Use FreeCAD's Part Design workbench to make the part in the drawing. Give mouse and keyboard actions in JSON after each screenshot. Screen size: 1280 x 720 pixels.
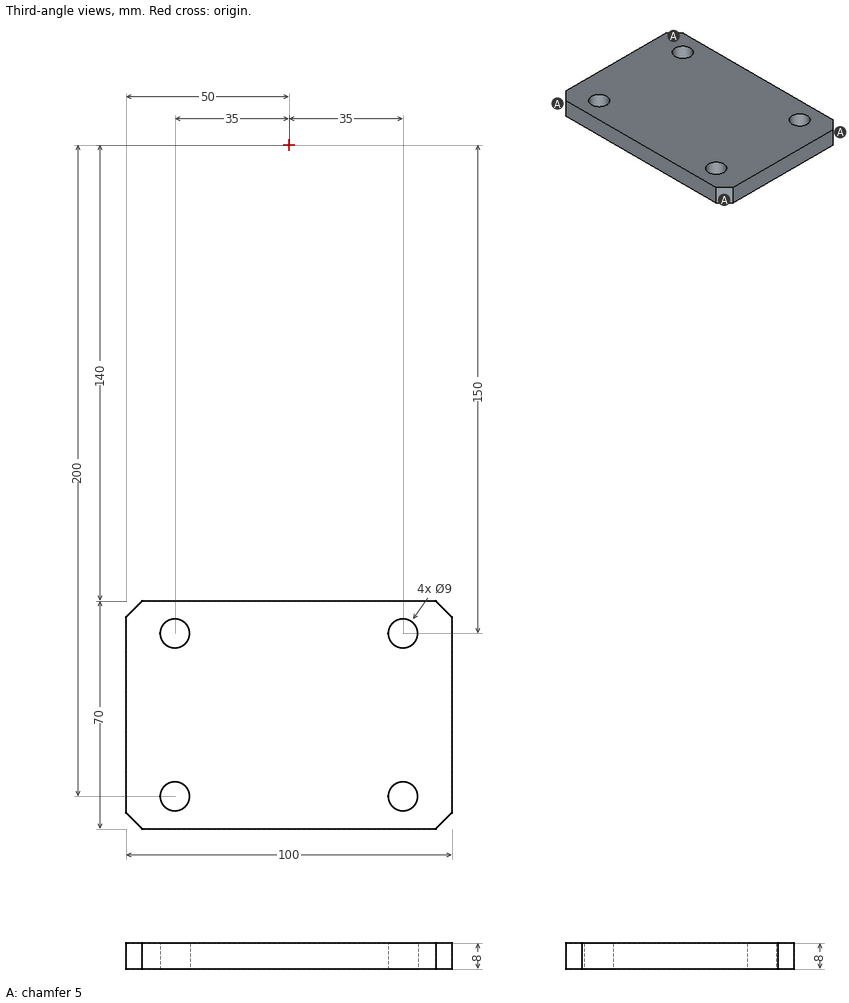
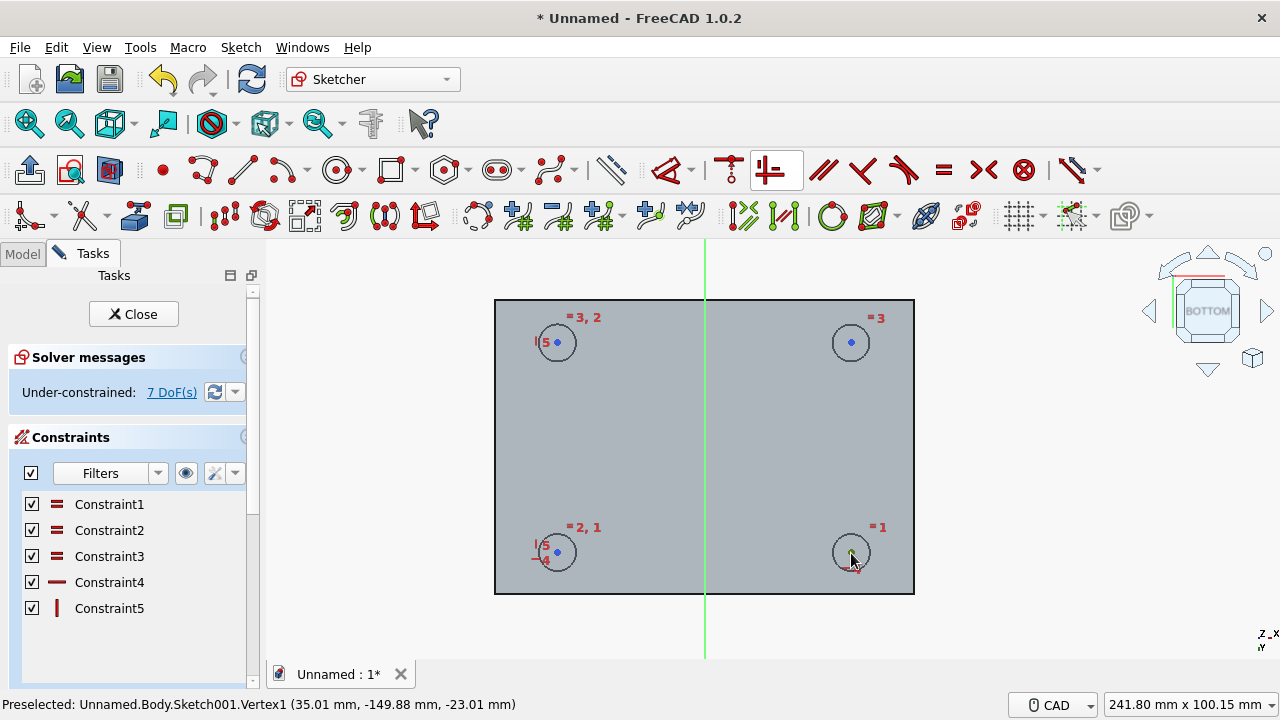
{"action": "left_click", "coordinate": [851, 343]}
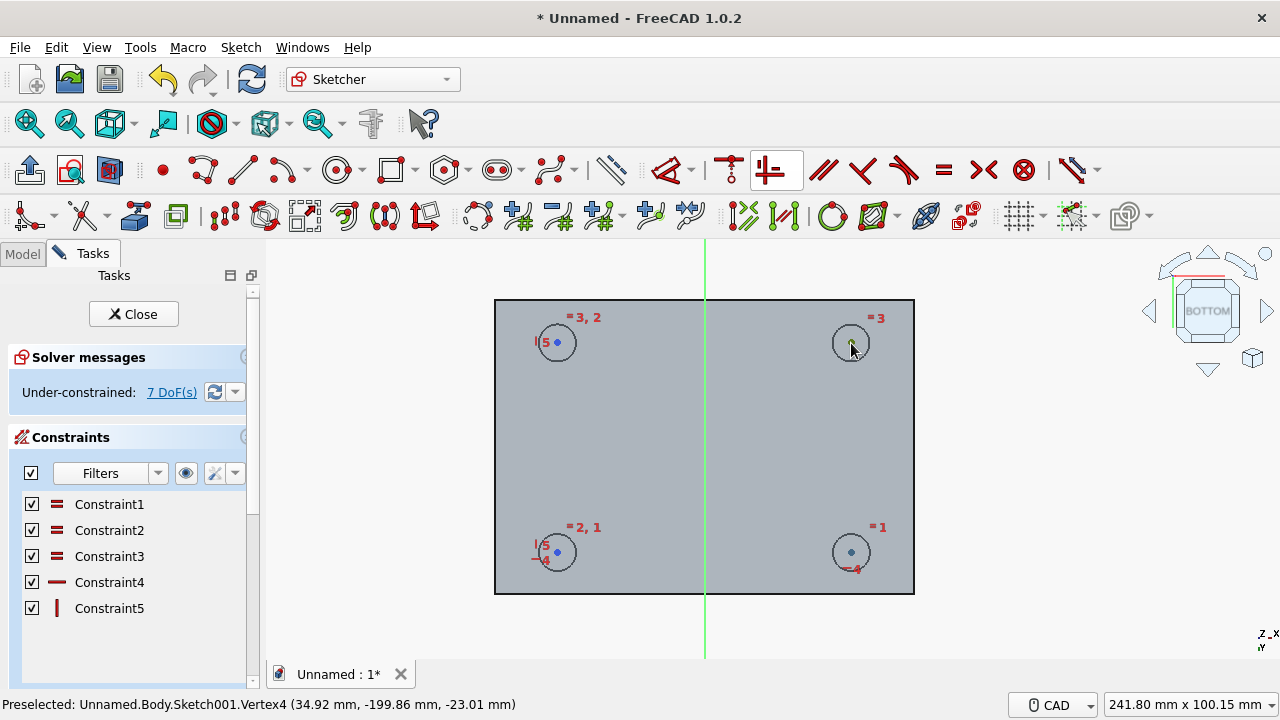
{"action": "left_click", "coordinate": [798, 170]}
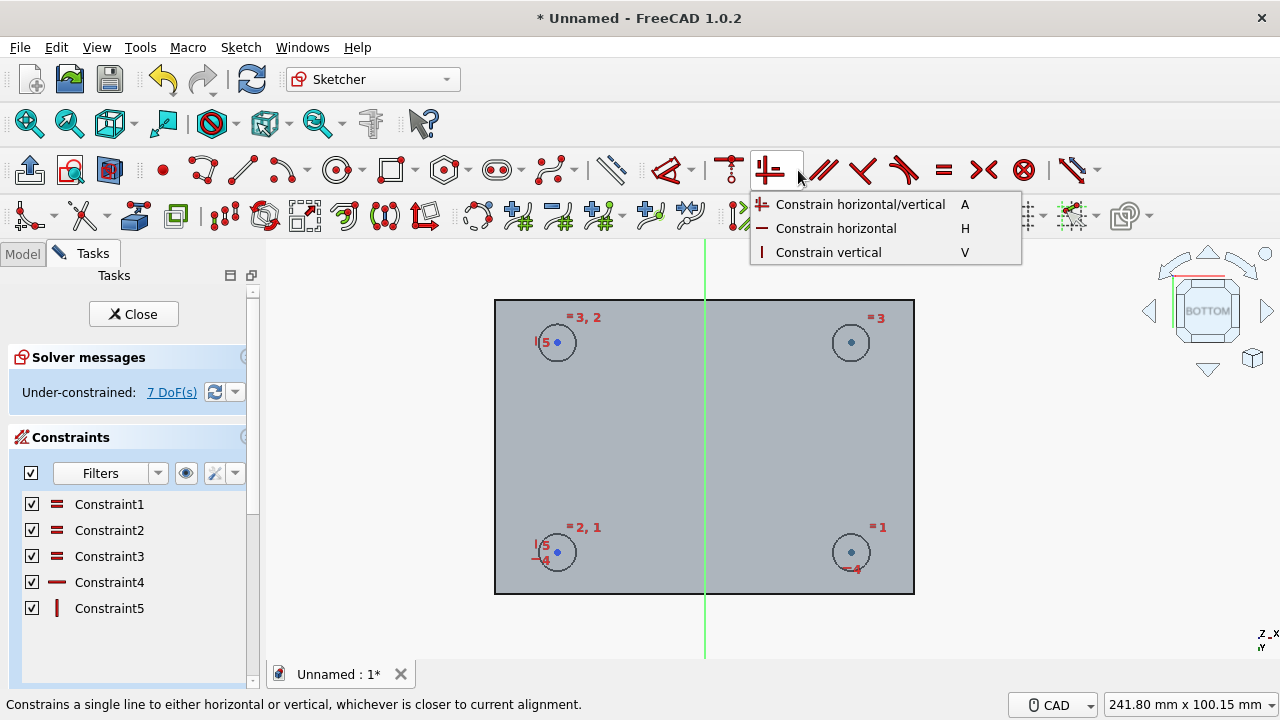
{"action": "left_click", "coordinate": [886, 252]}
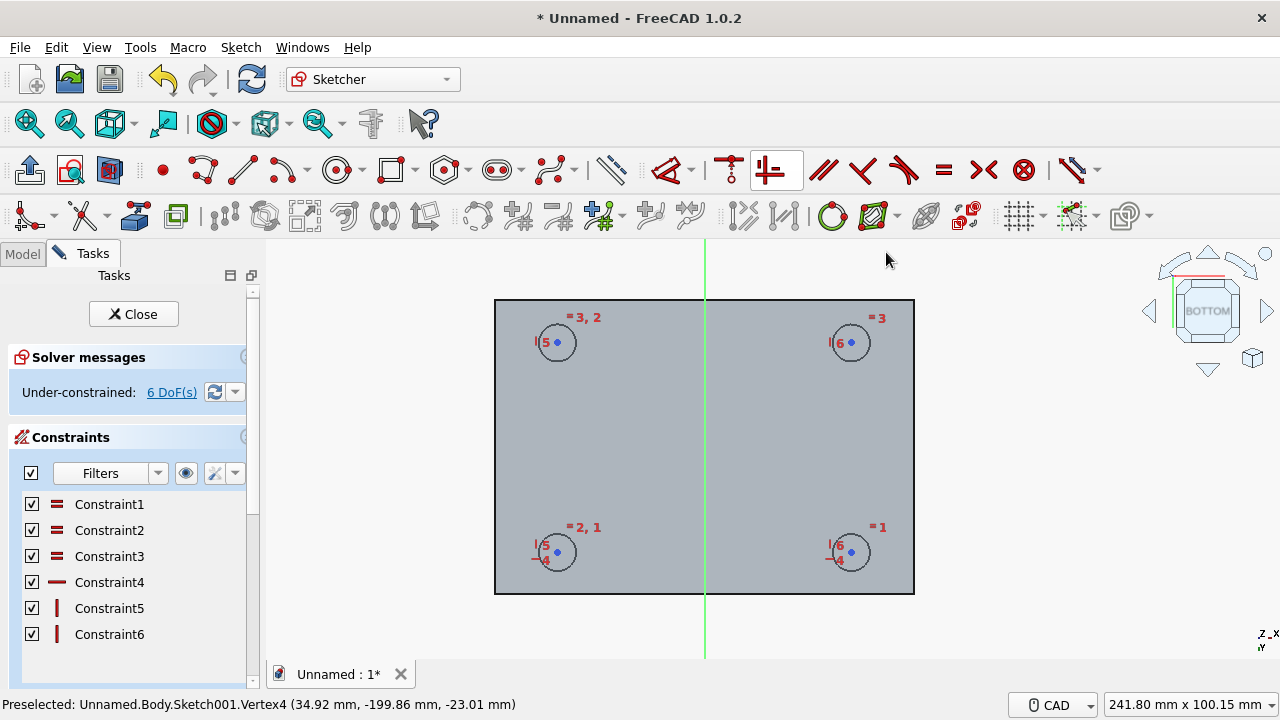
{"action": "left_click", "coordinate": [557, 343]}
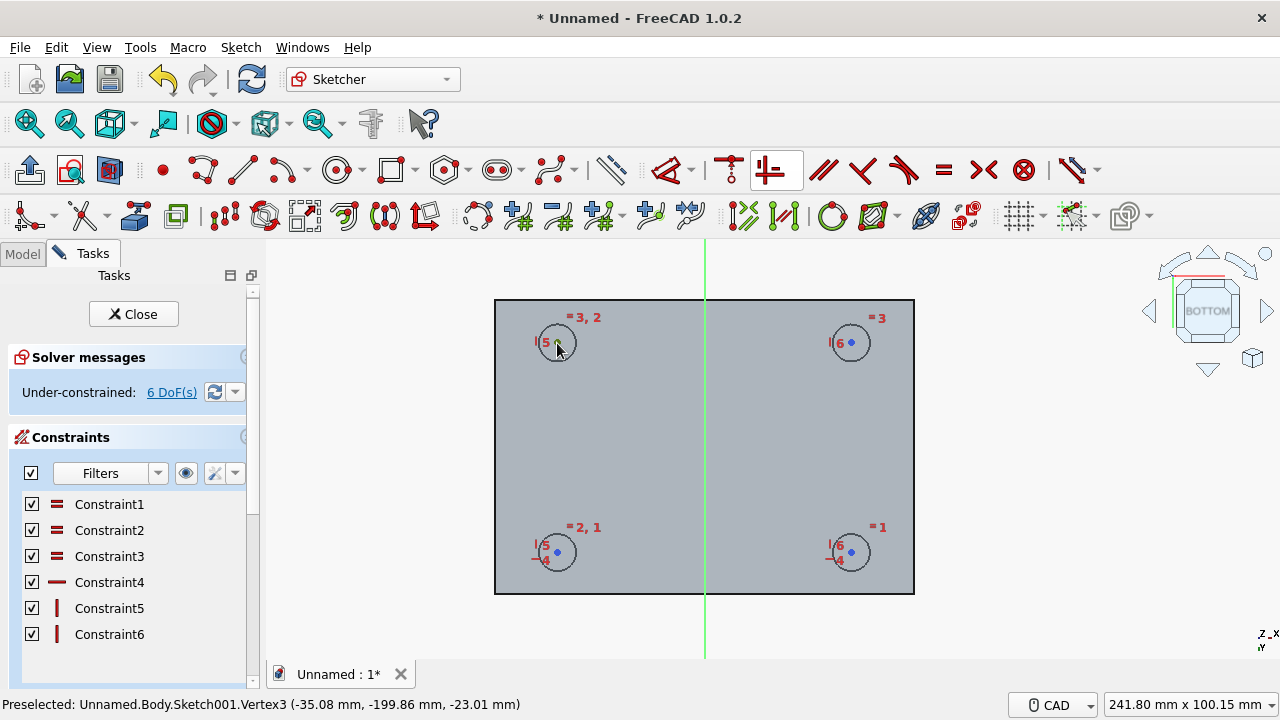
{"action": "left_click", "coordinate": [851, 343]}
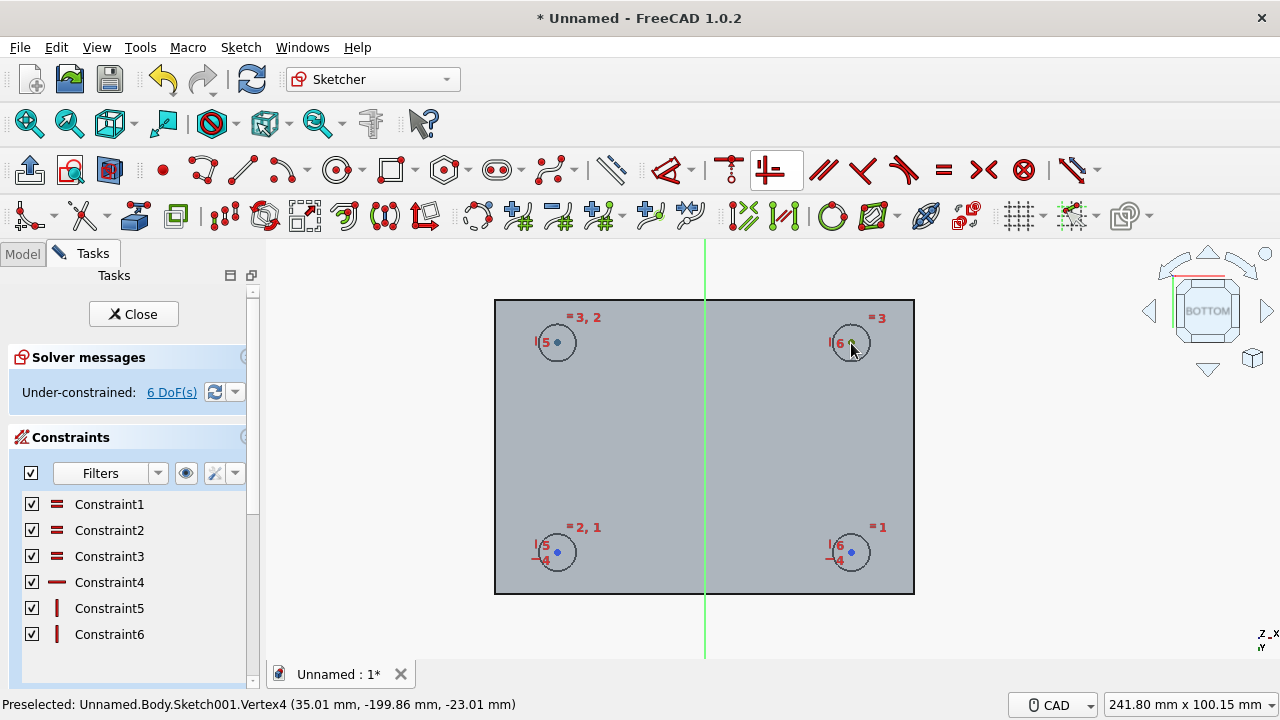
{"action": "left_click", "coordinate": [798, 170]}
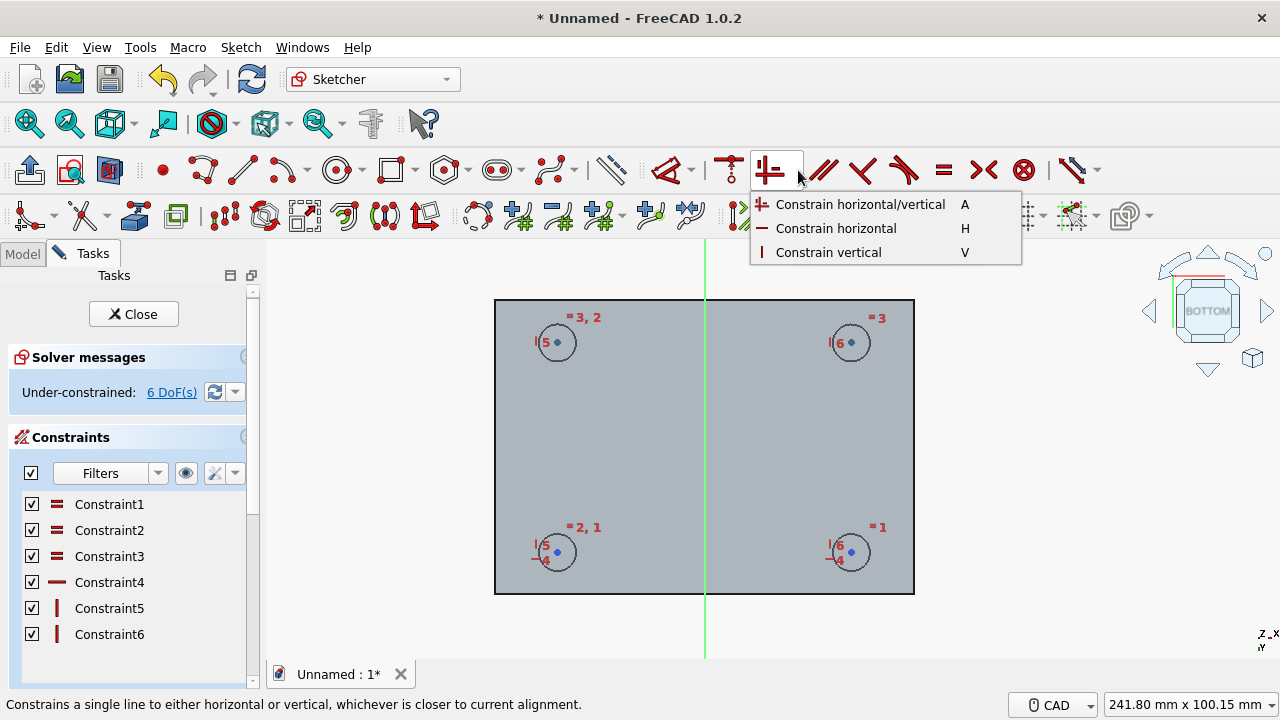
{"action": "left_click", "coordinate": [886, 228]}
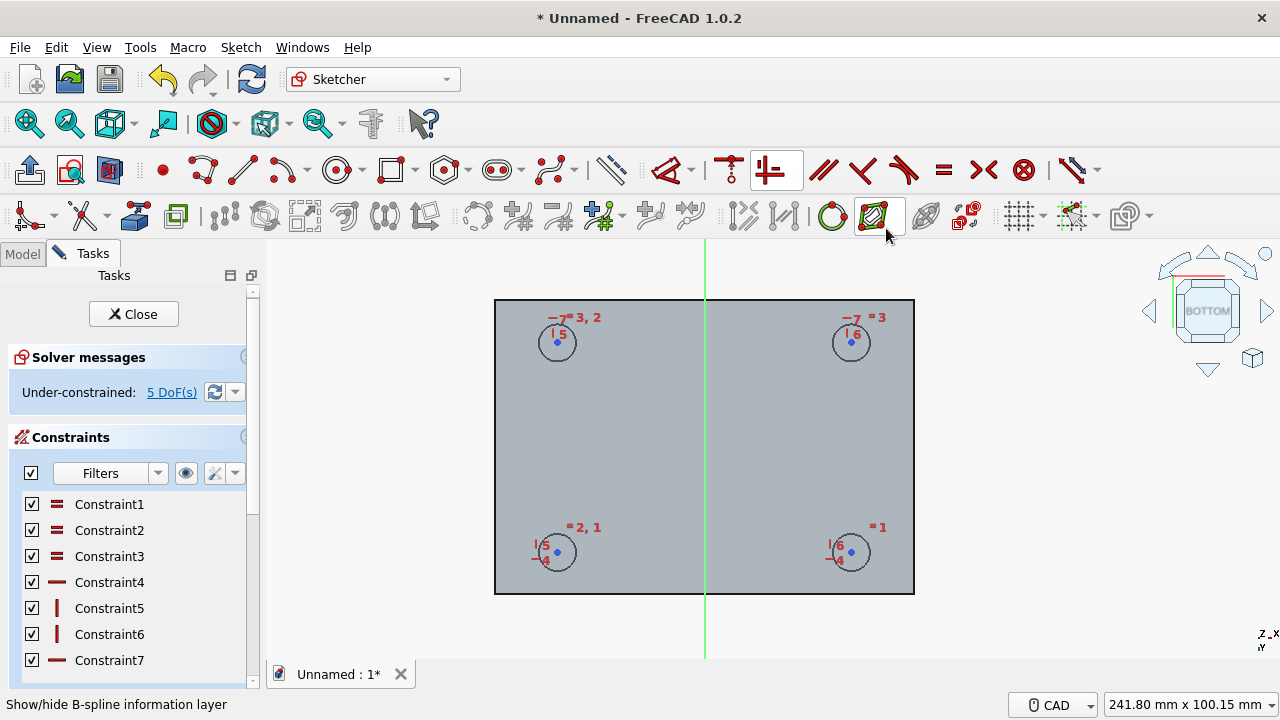
{"action": "left_click", "coordinate": [666, 170]}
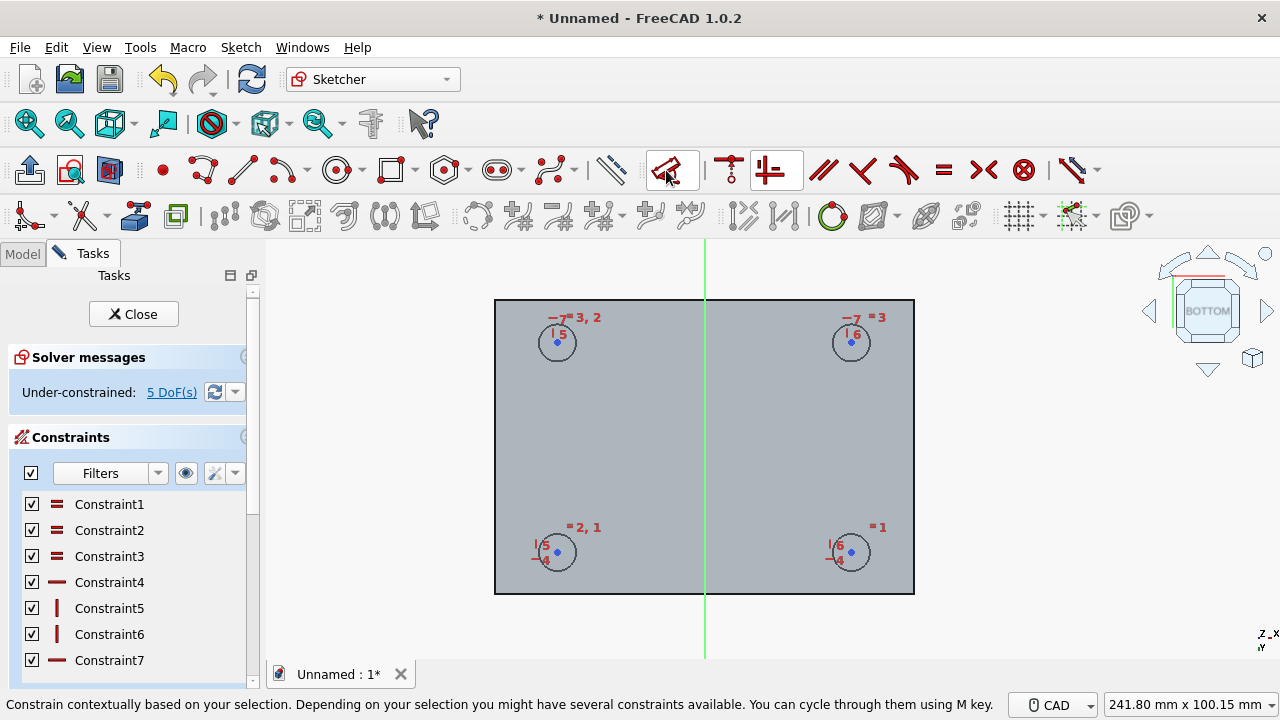
{"action": "left_click", "coordinate": [864, 539]}
{"action": "left_click", "coordinate": [886, 516]}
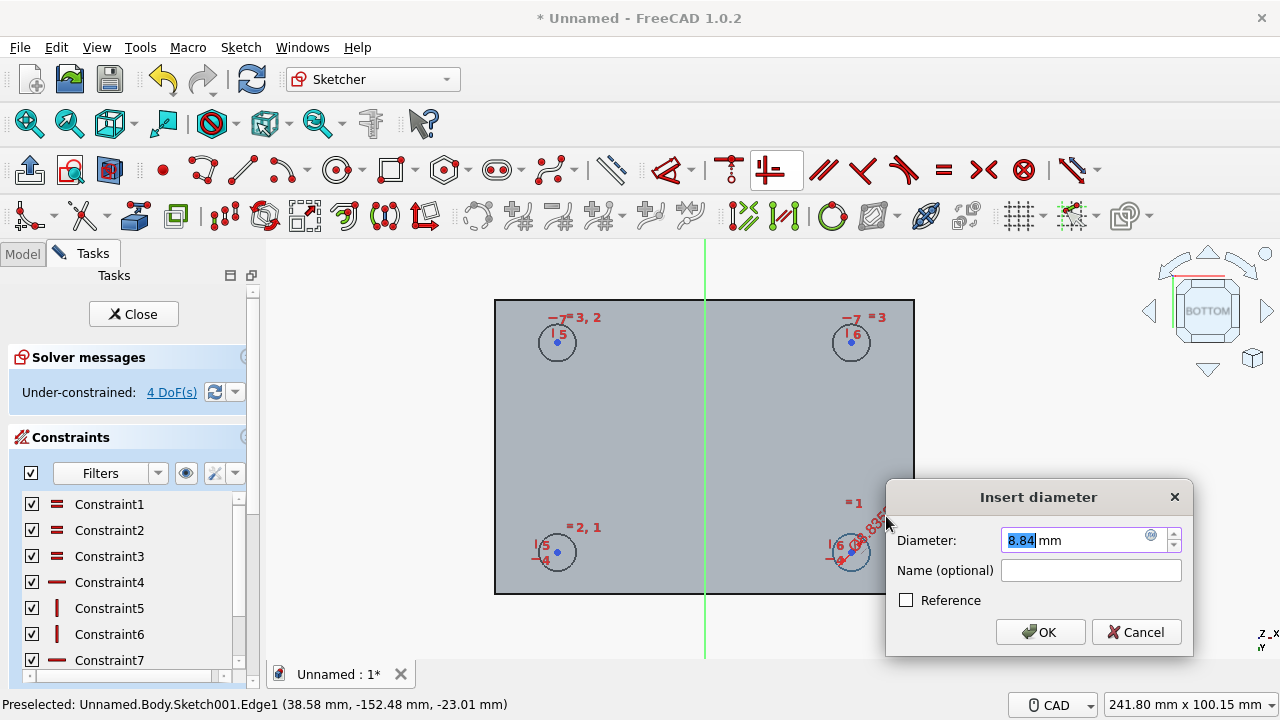
{"action": "type", "text": "9"}
{"action": "key", "text": "Return"}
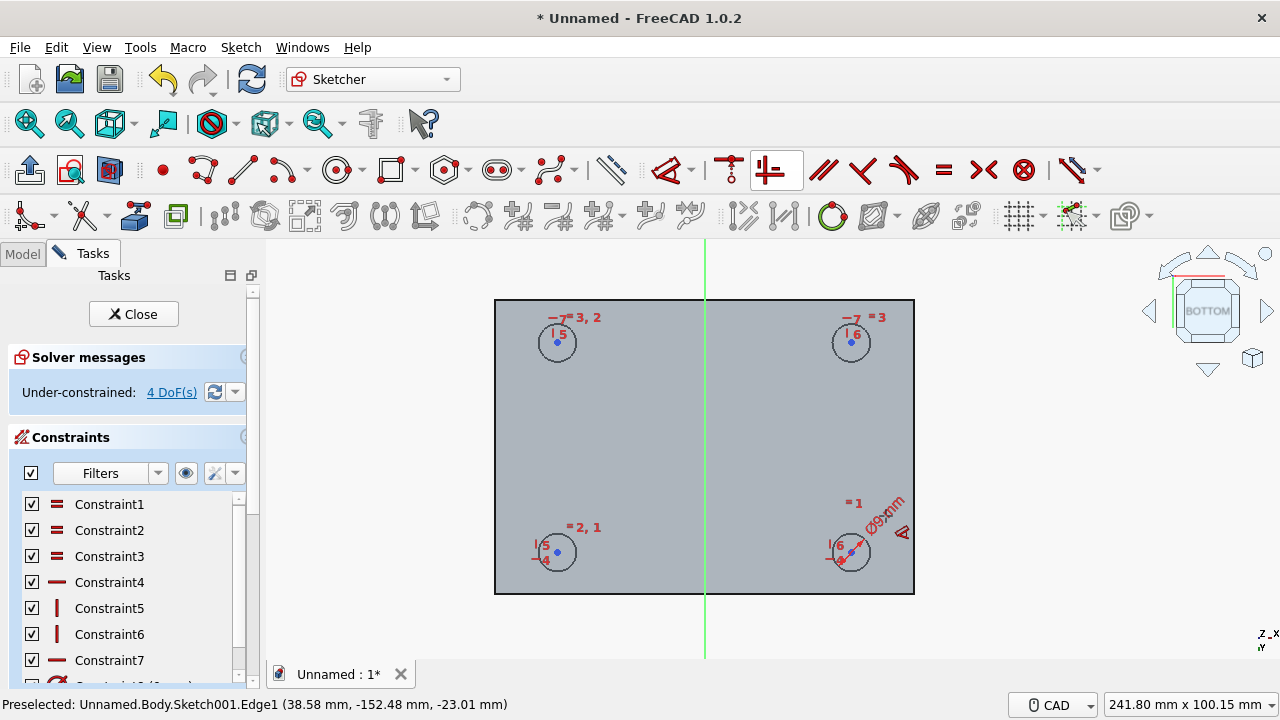
{"action": "left_click", "coordinate": [851, 553]}
{"action": "left_click", "coordinate": [778, 519]}